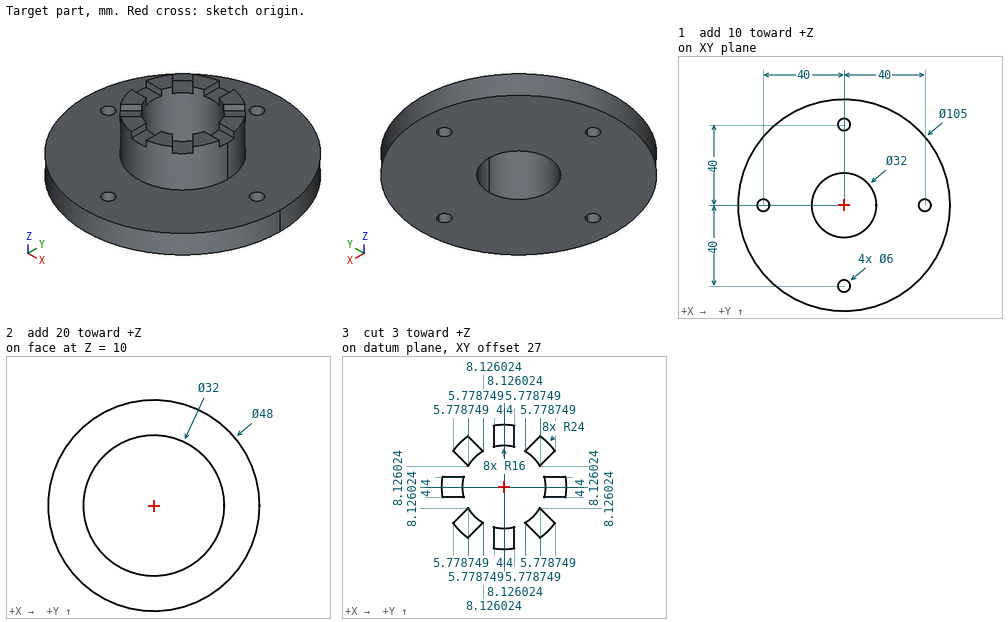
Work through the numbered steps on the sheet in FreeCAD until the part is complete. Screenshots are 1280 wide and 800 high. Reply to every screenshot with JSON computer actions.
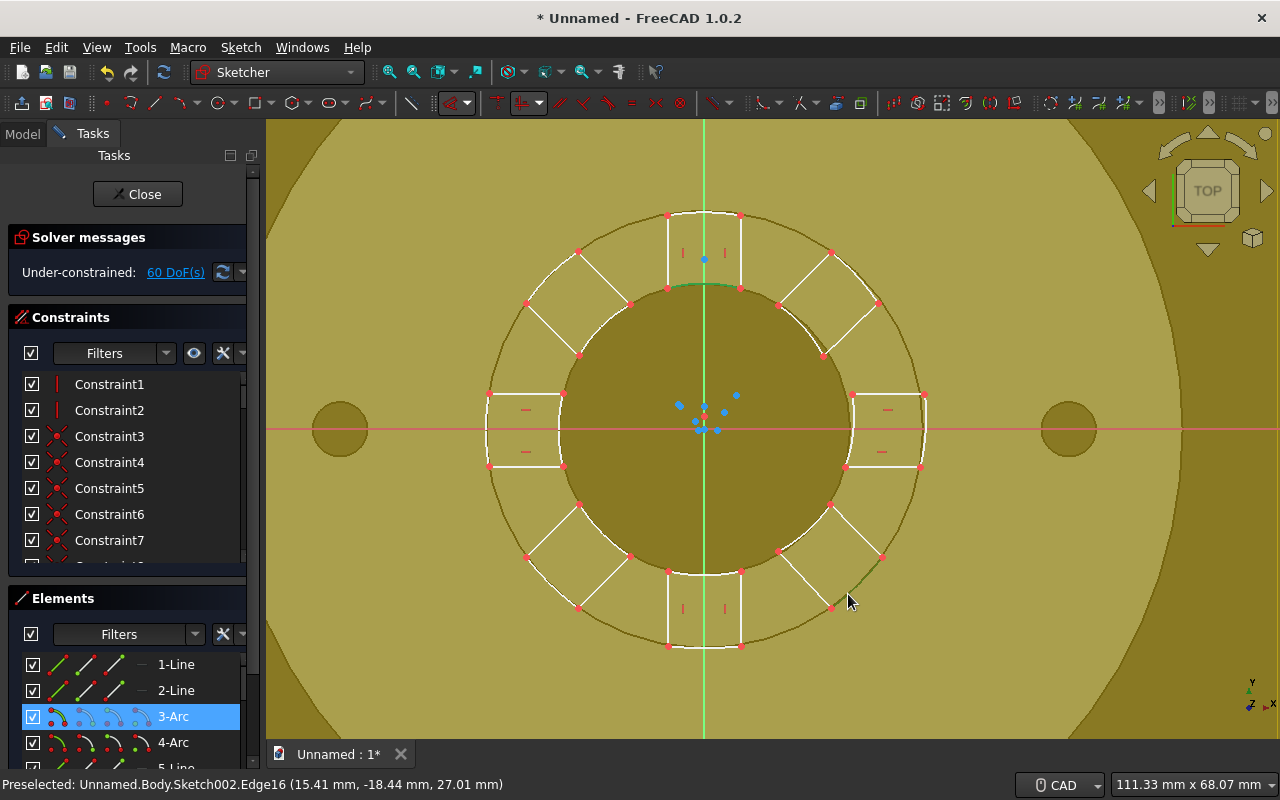
{"action": "left_click", "coordinate": [498, 104]}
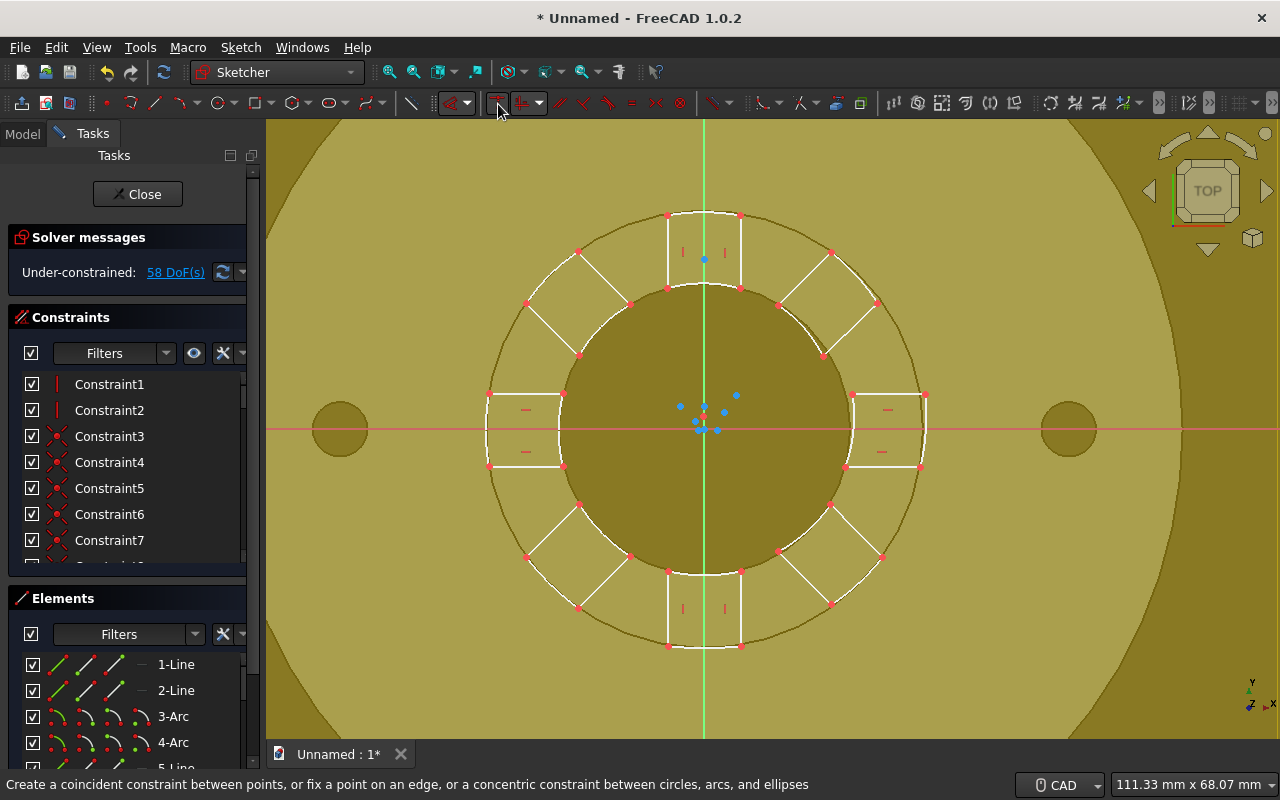
{"action": "left_click", "coordinate": [719, 284]}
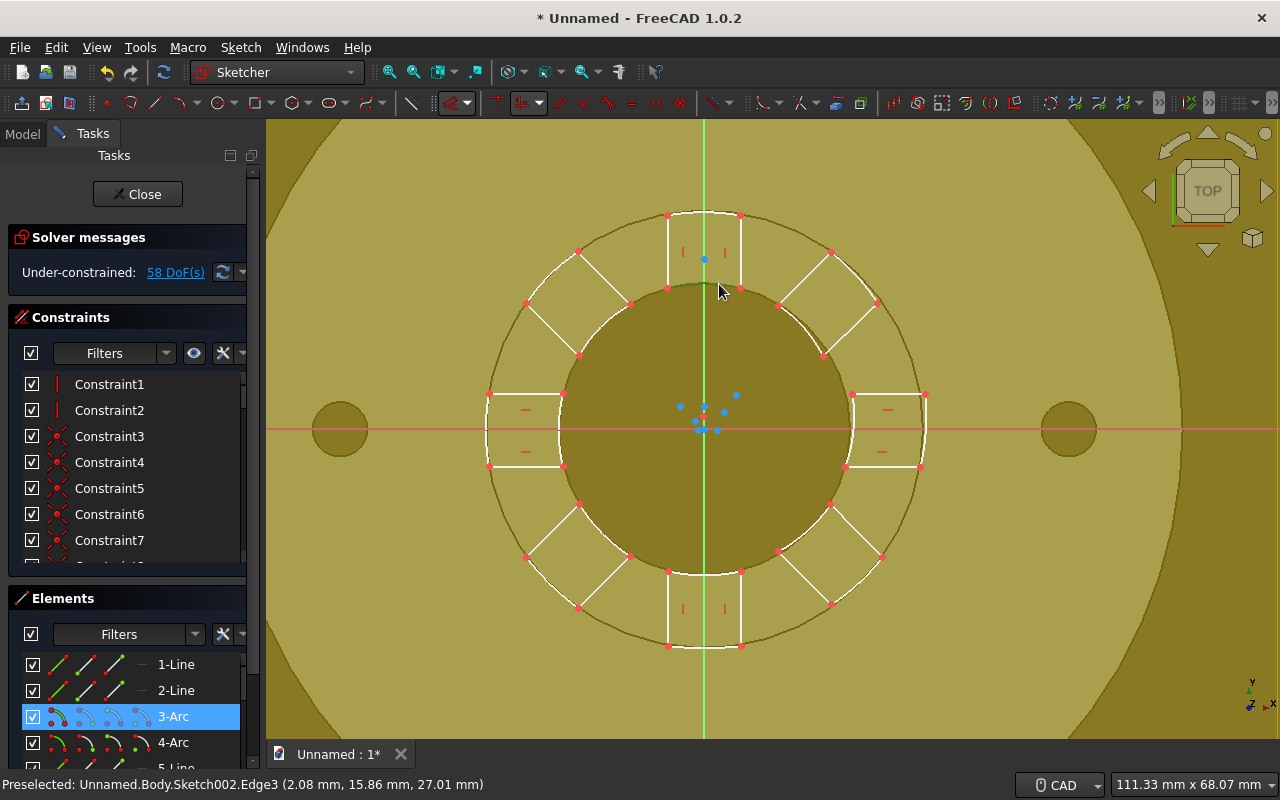
{"action": "left_click", "coordinate": [690, 575]}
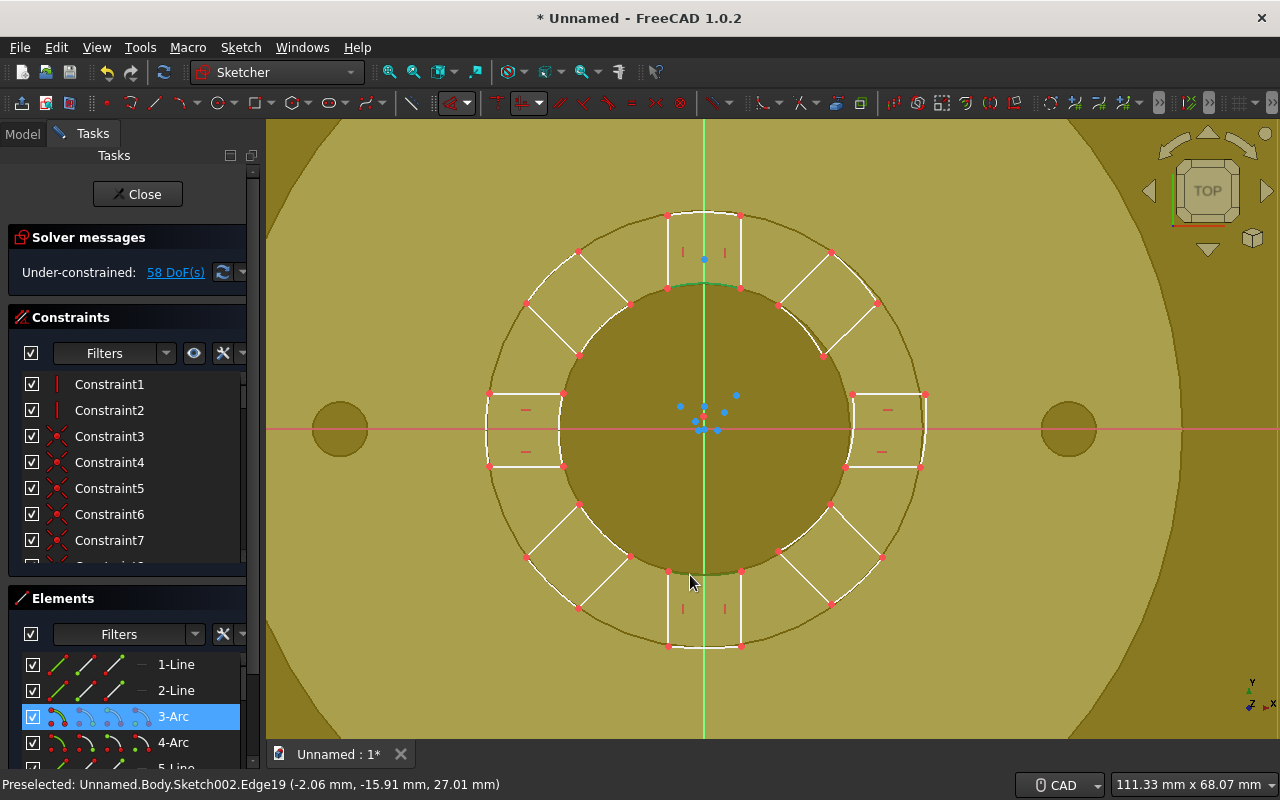
{"action": "left_click", "coordinate": [498, 104]}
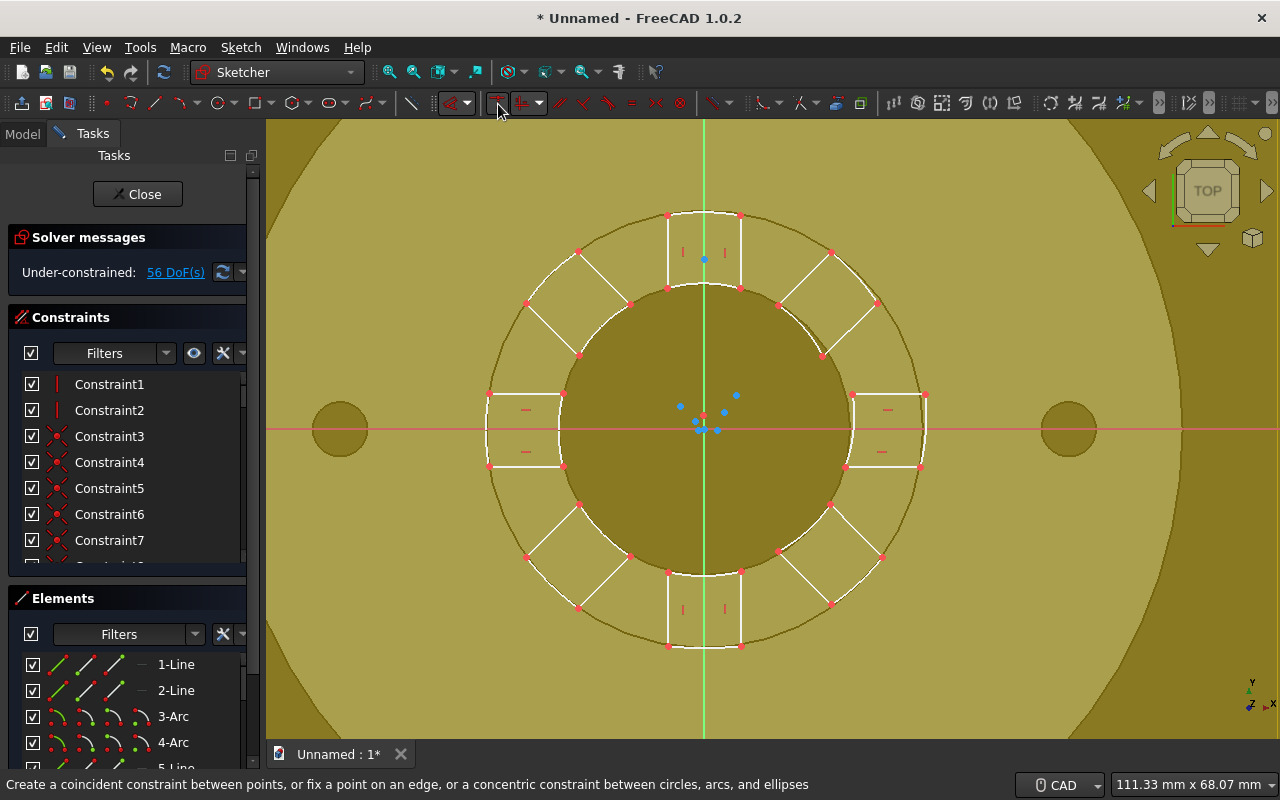
{"action": "left_click", "coordinate": [719, 284]}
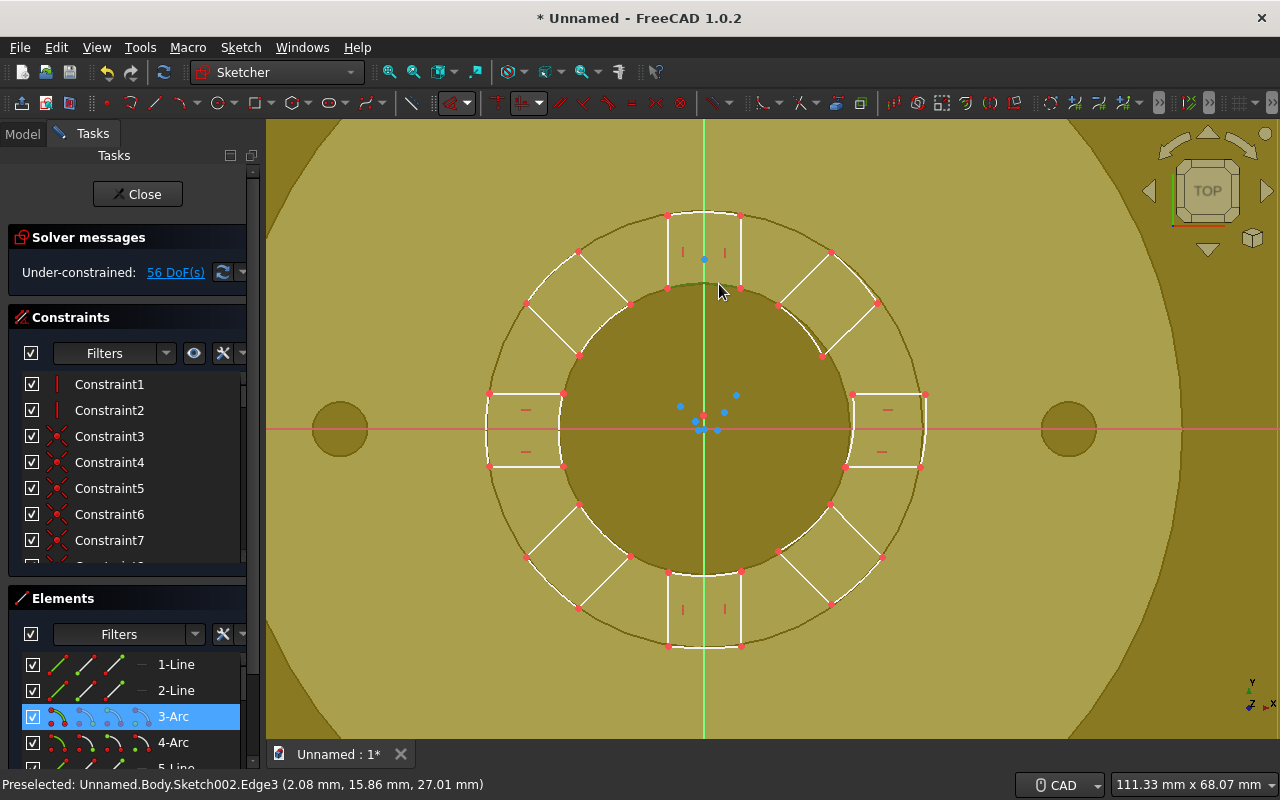
{"action": "left_click", "coordinate": [690, 648]}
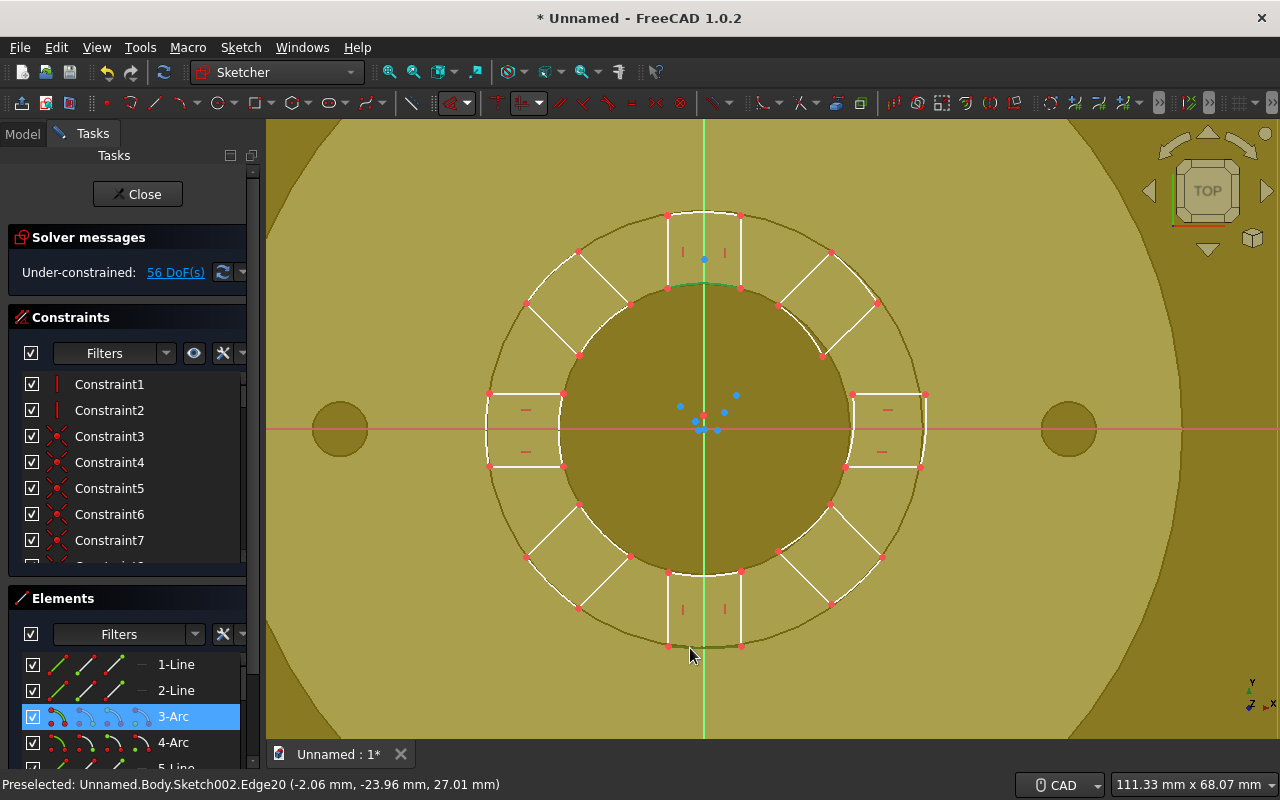
{"action": "left_click", "coordinate": [498, 104]}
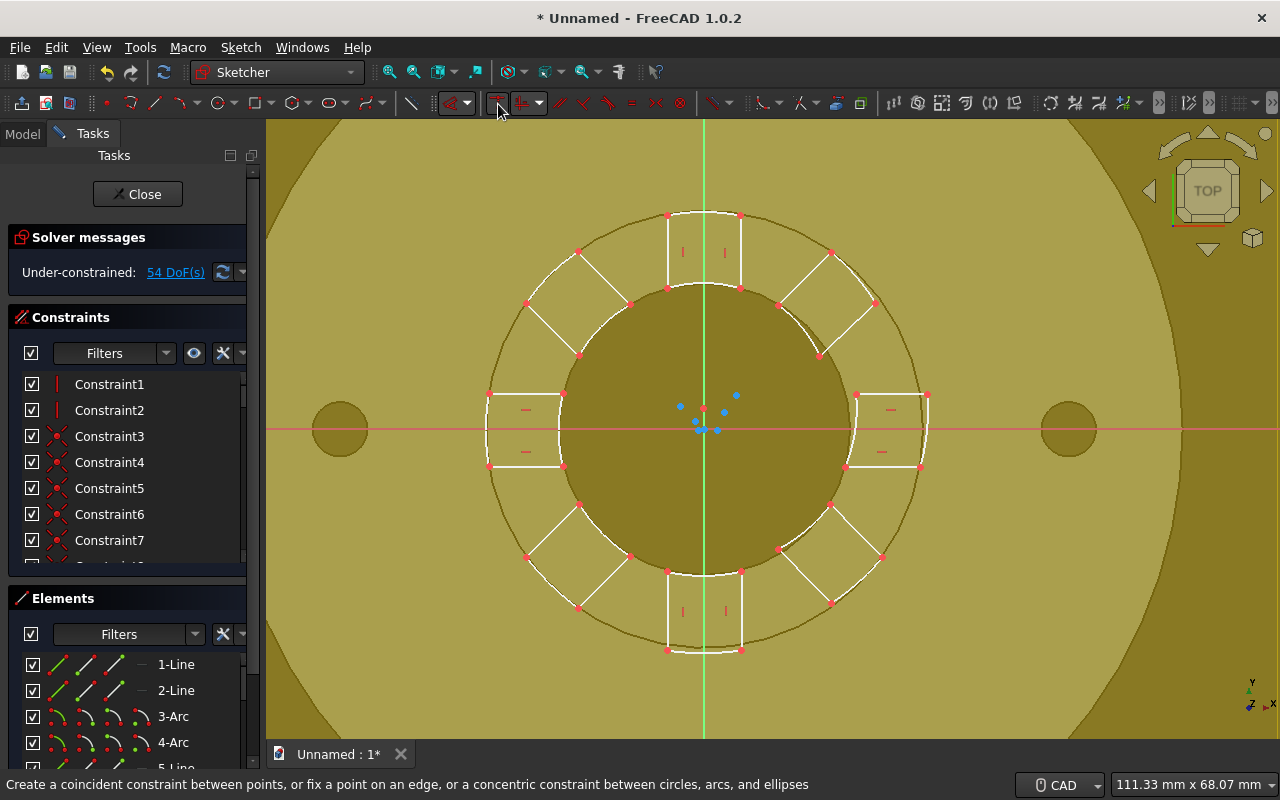
{"action": "left_click", "coordinate": [719, 284]}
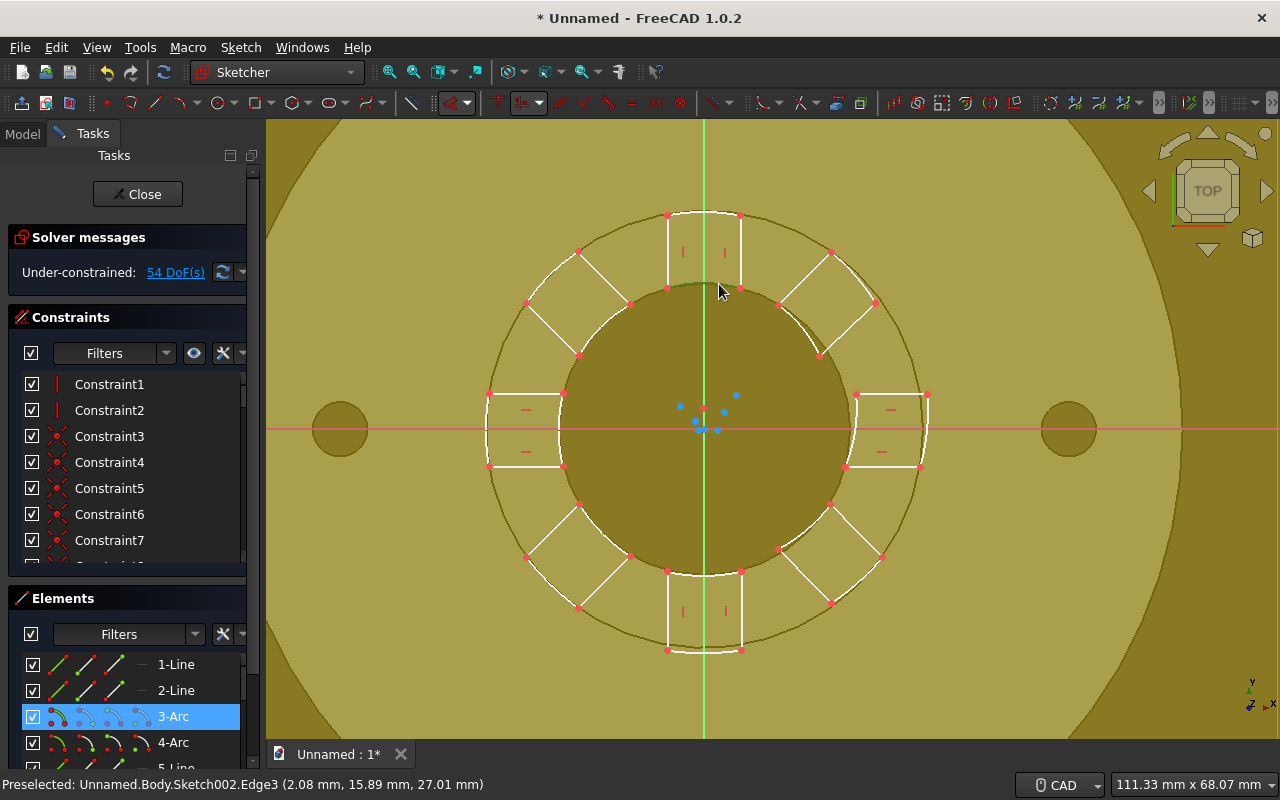
{"action": "left_click", "coordinate": [592, 522]}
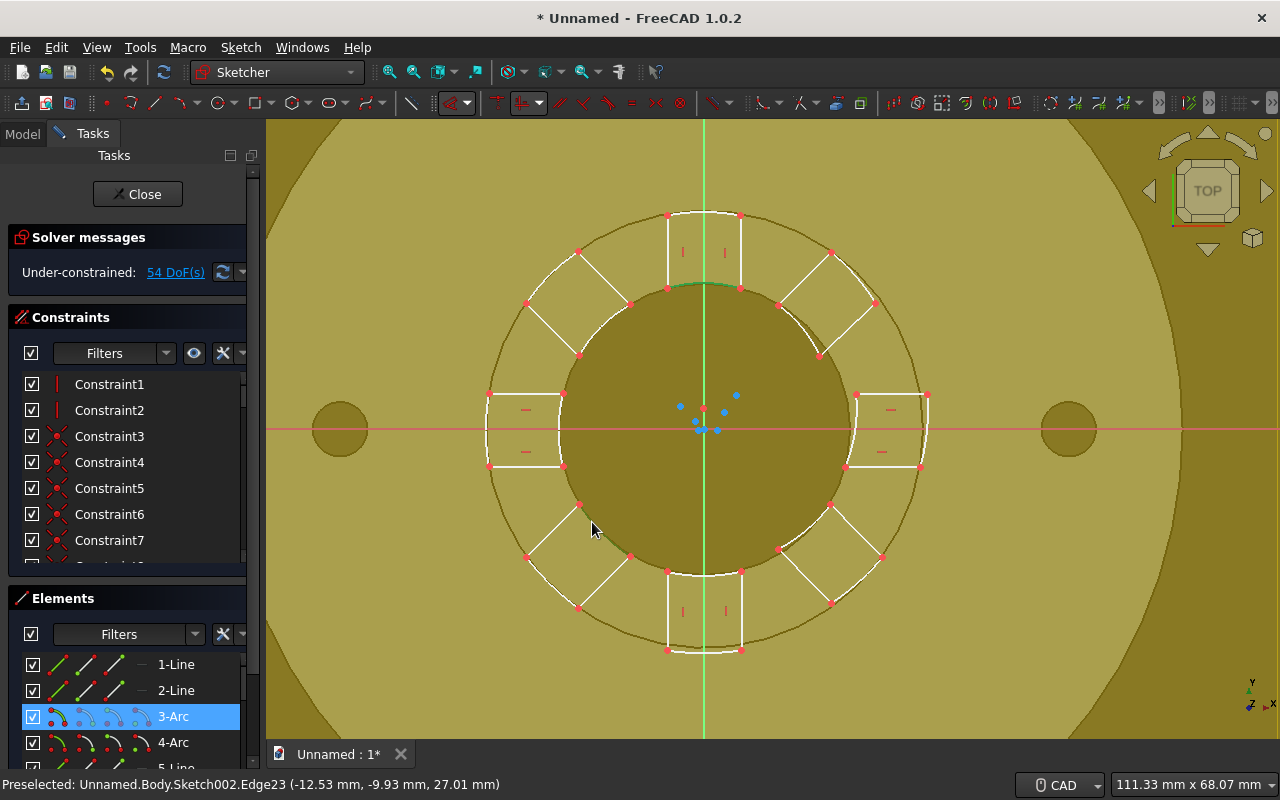
{"action": "left_click", "coordinate": [498, 104]}